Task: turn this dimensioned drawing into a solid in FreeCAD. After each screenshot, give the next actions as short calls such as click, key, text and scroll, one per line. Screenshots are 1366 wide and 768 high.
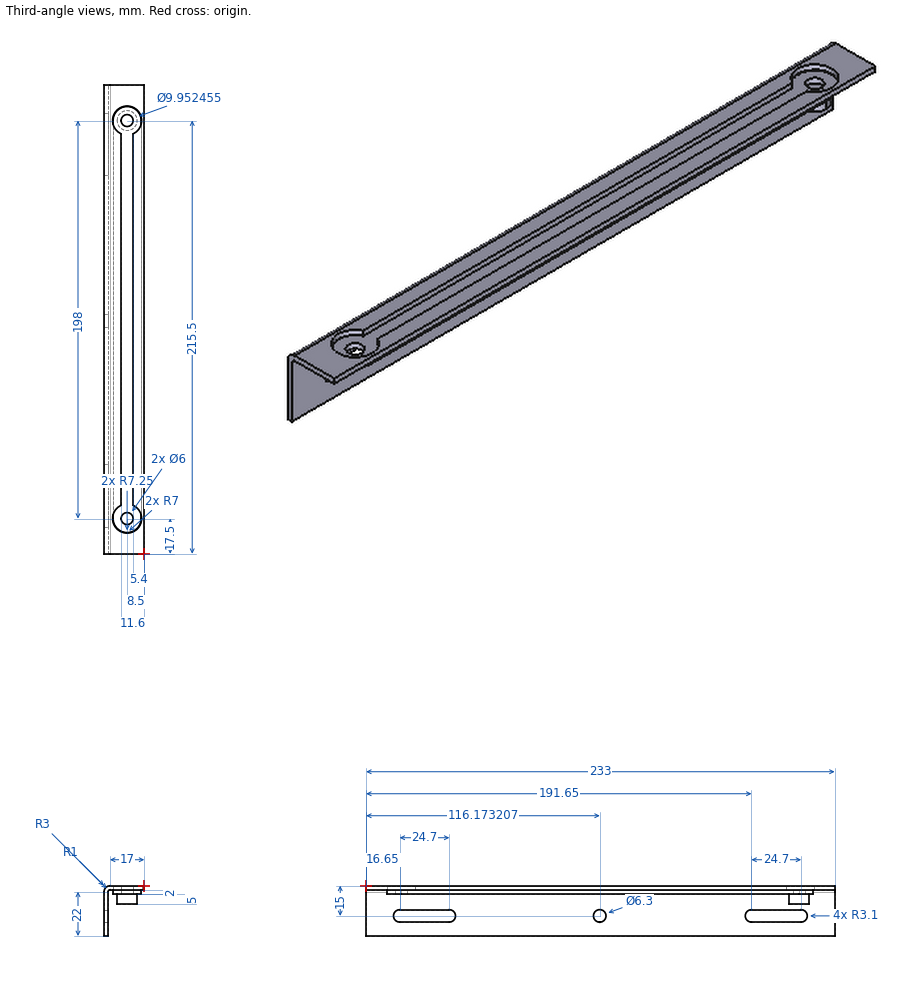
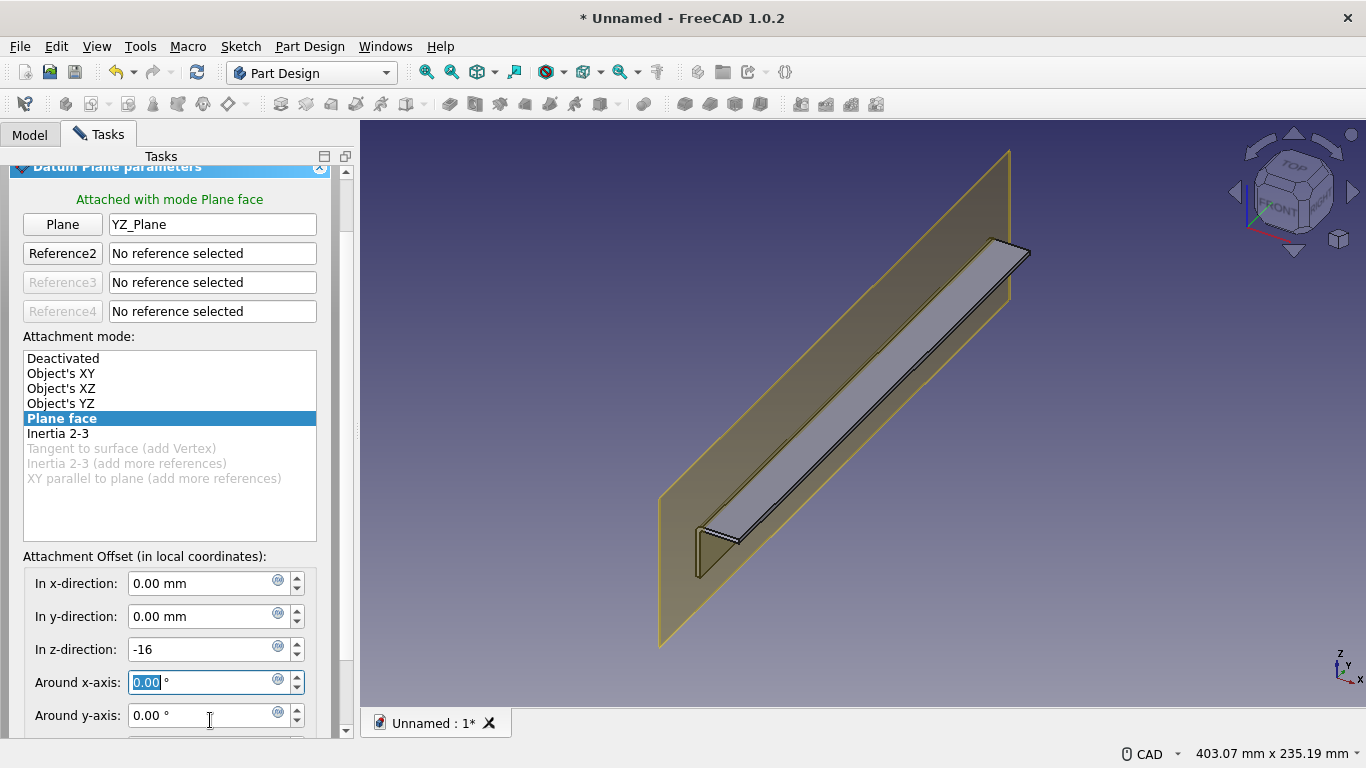
scroll(346, 452, up, 2)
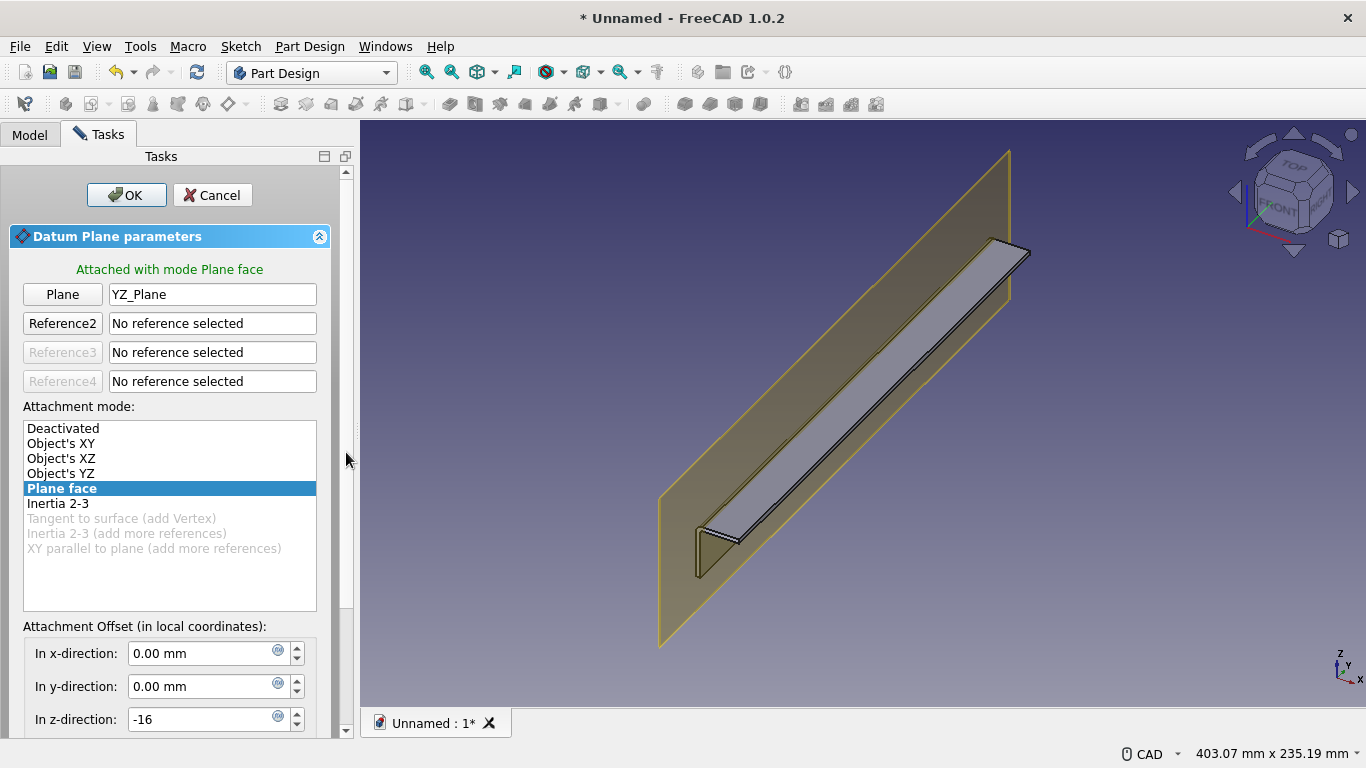
click(127, 195)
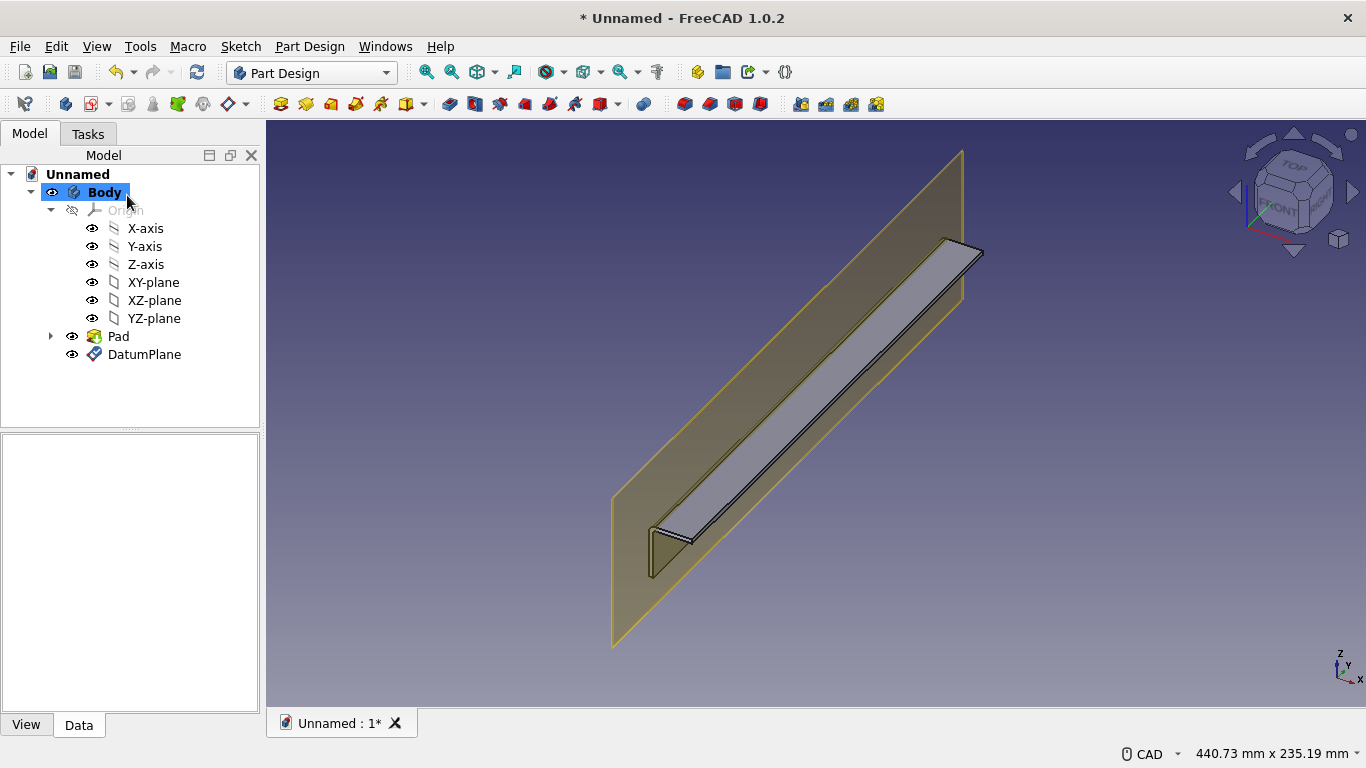
click(117, 354)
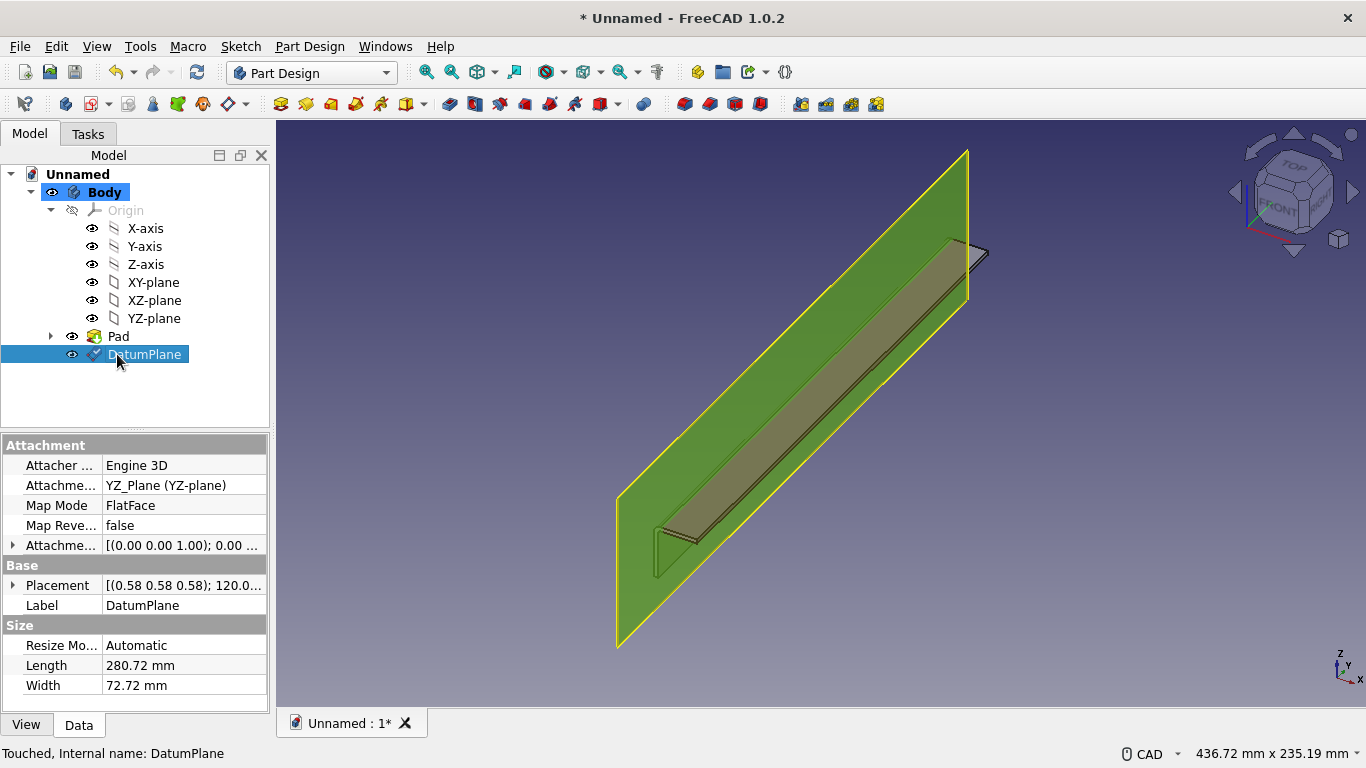
click(90, 104)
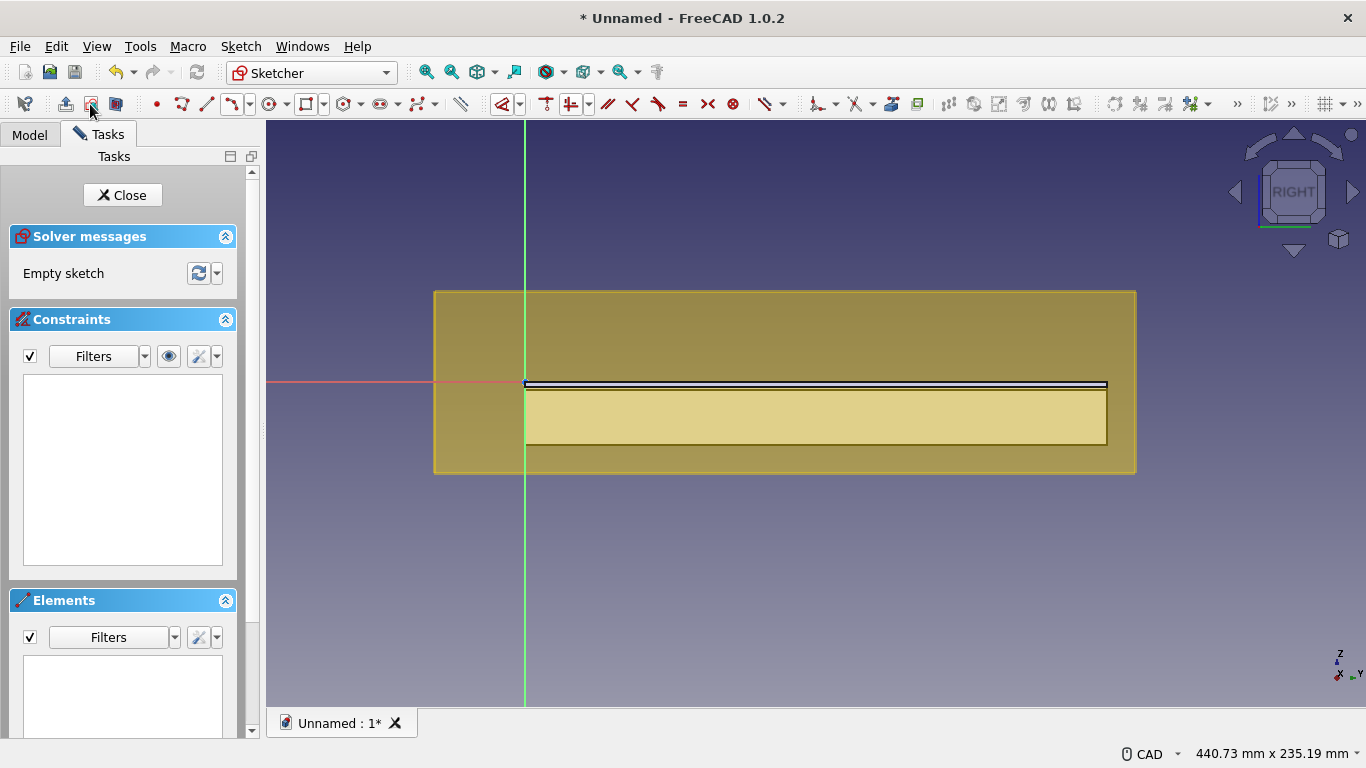
click(116, 104)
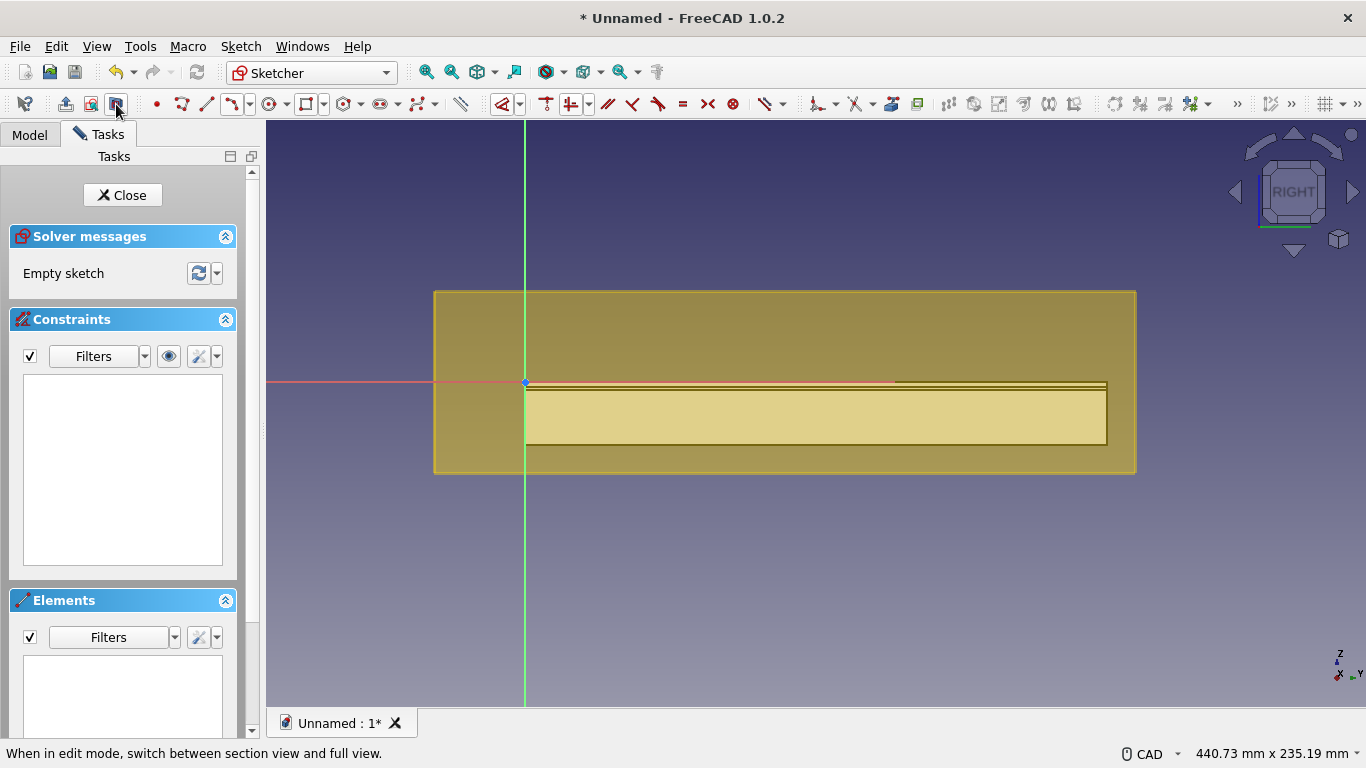
click(380, 104)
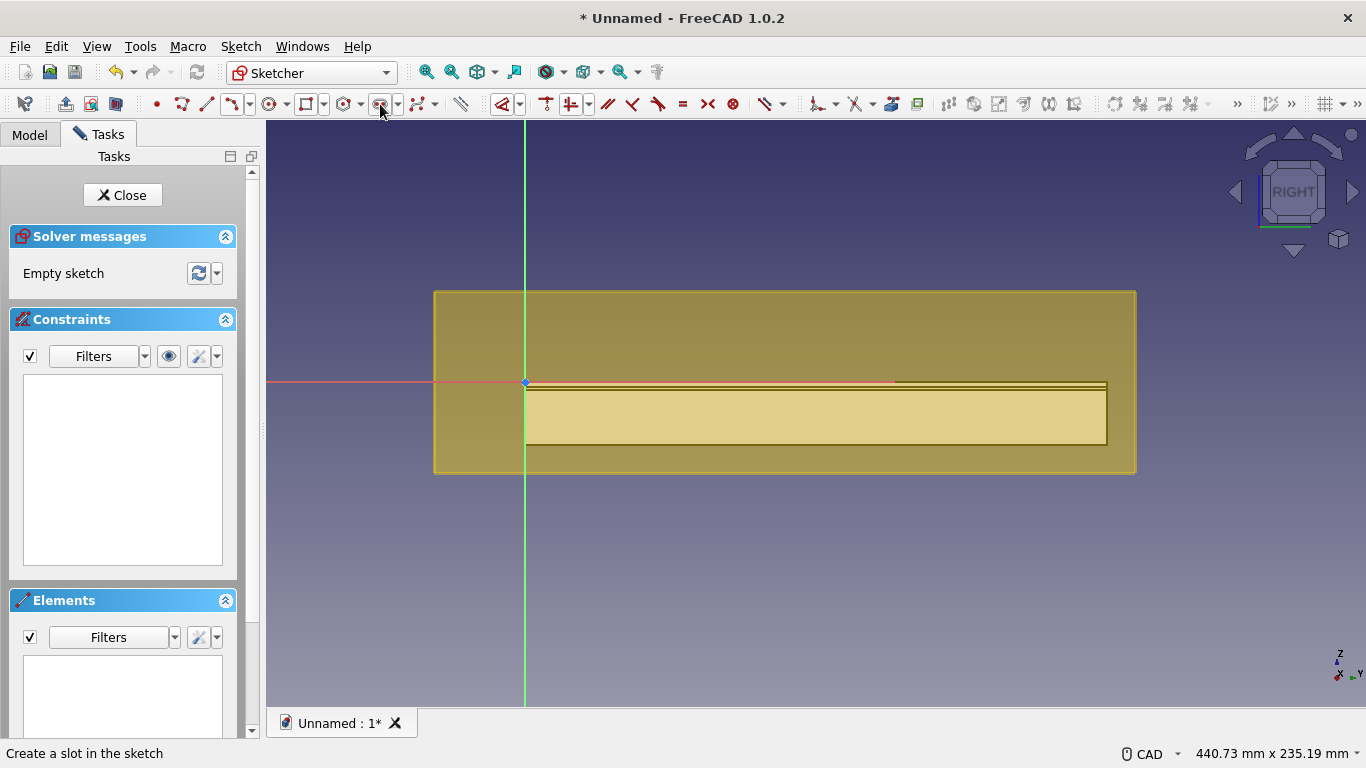
scroll(1004, 420, up, 6)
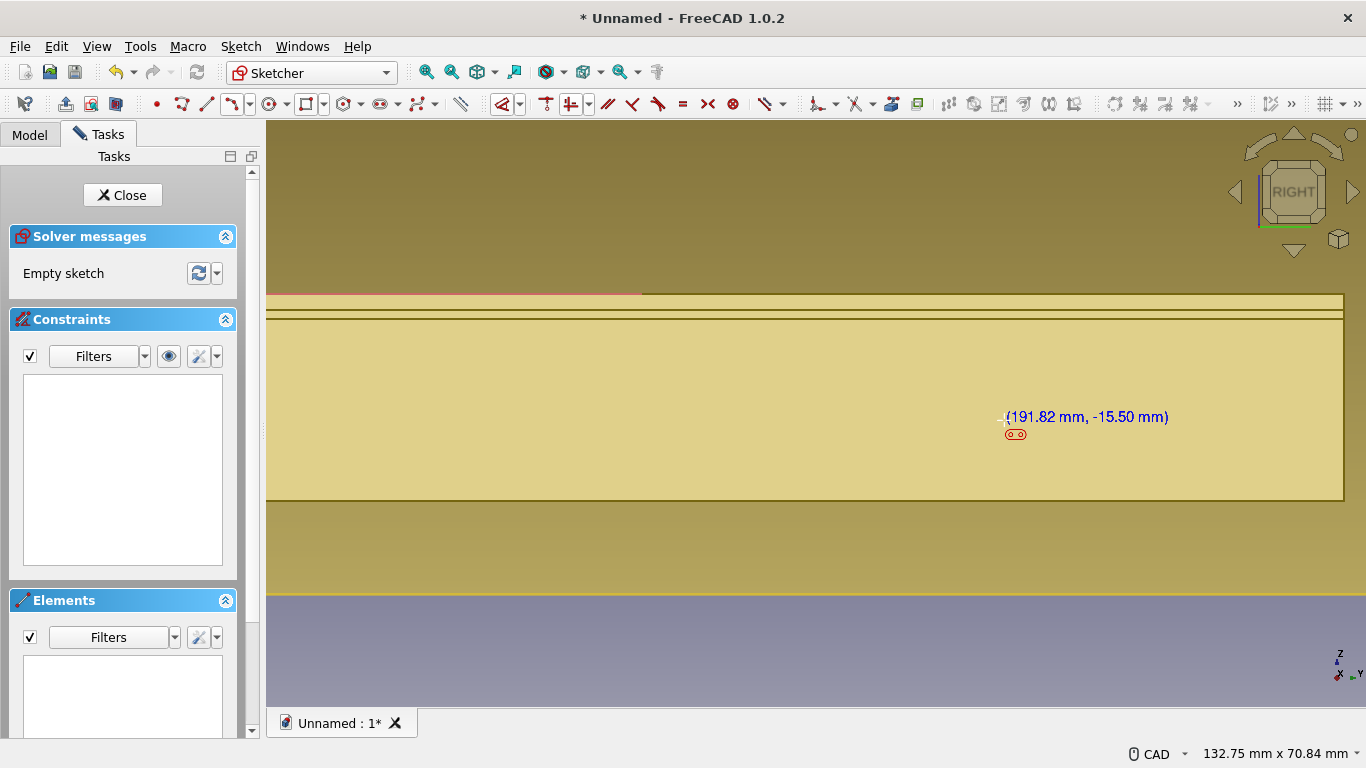
click(1001, 418)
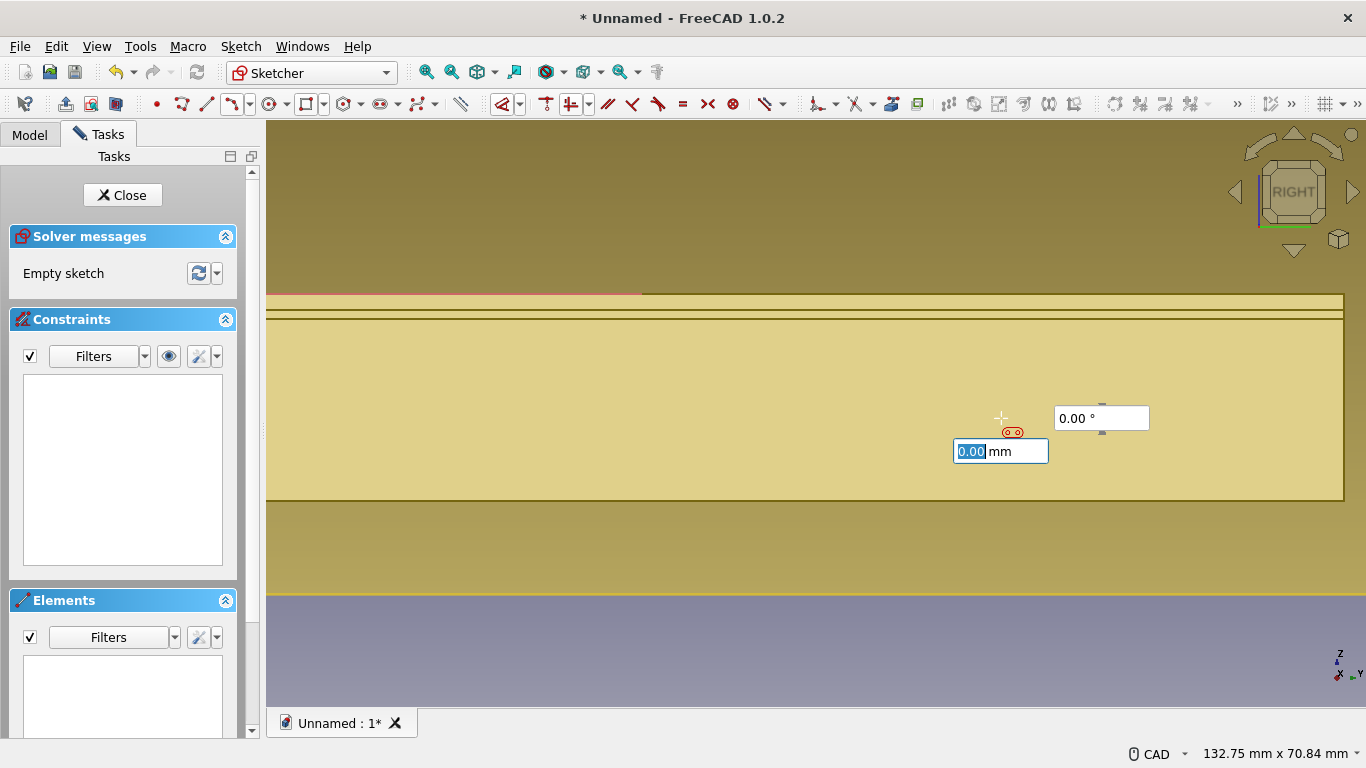
scroll(995, 439, down, 5)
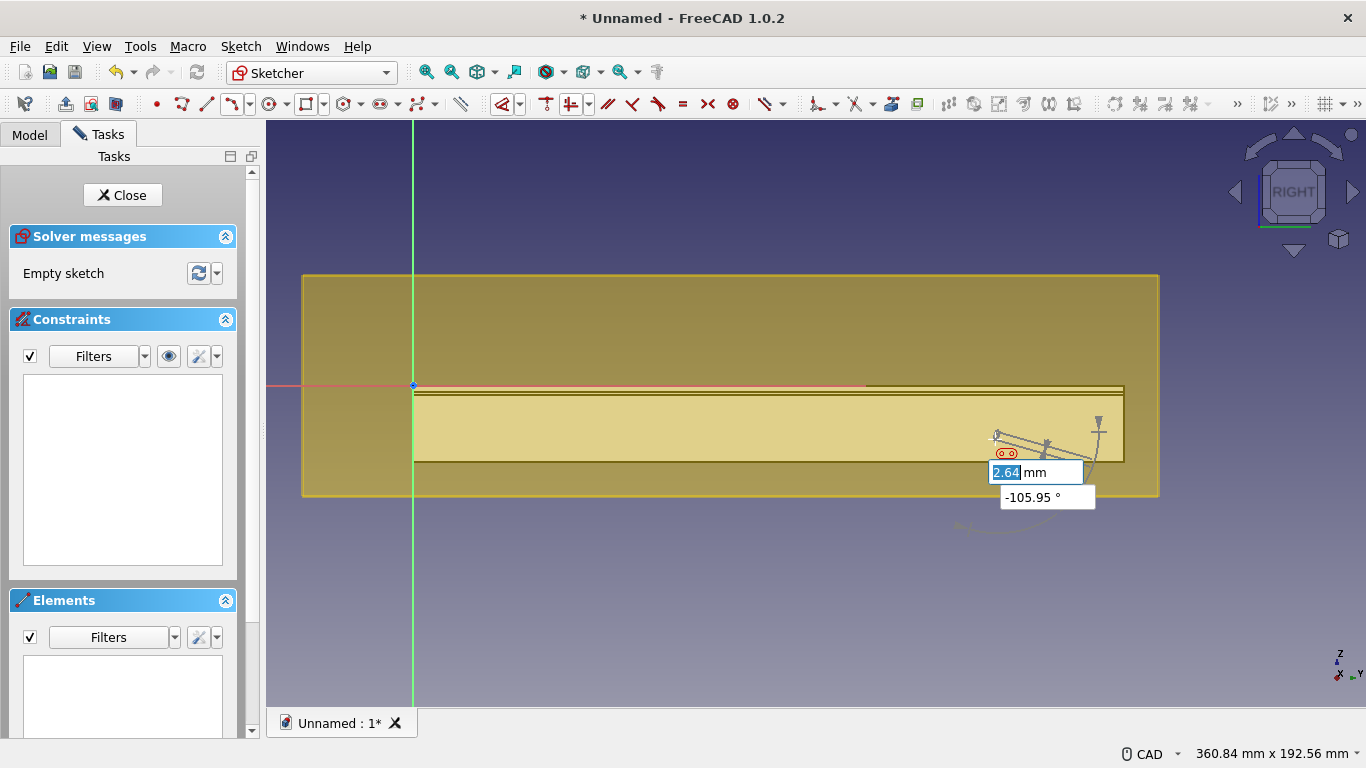
click(1073, 432)